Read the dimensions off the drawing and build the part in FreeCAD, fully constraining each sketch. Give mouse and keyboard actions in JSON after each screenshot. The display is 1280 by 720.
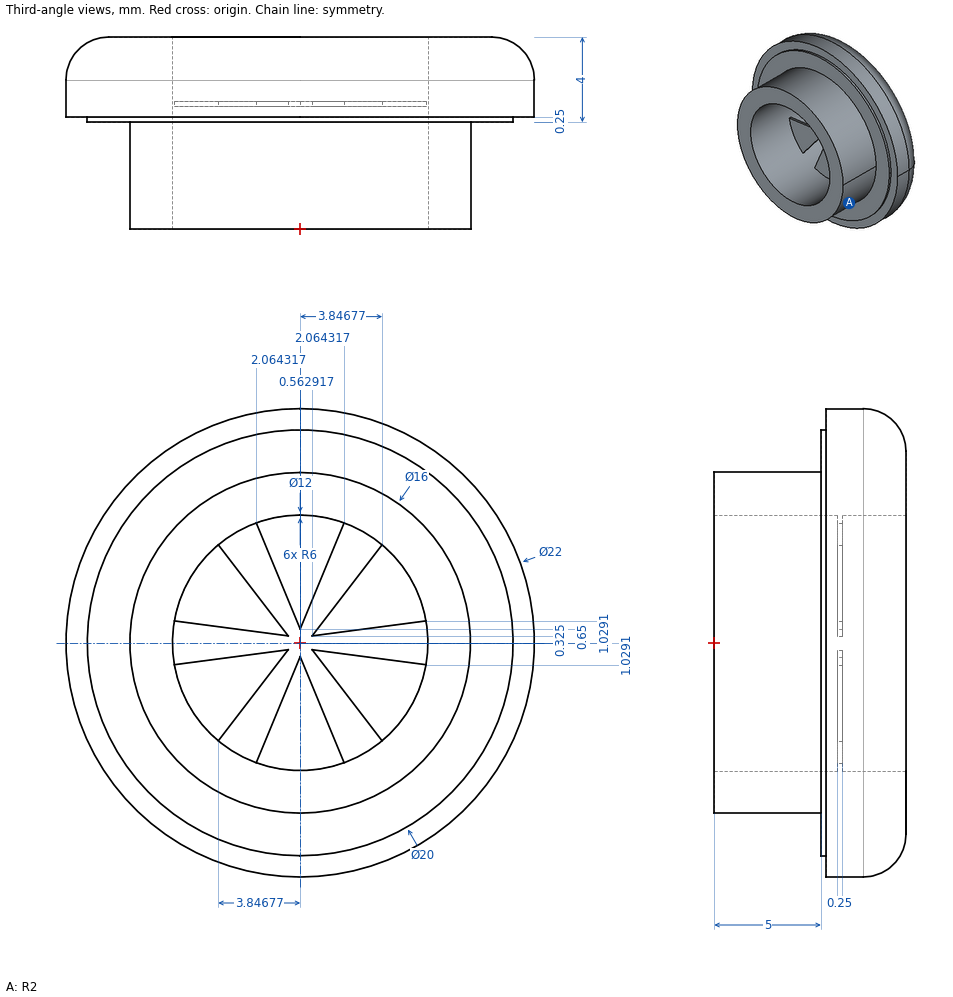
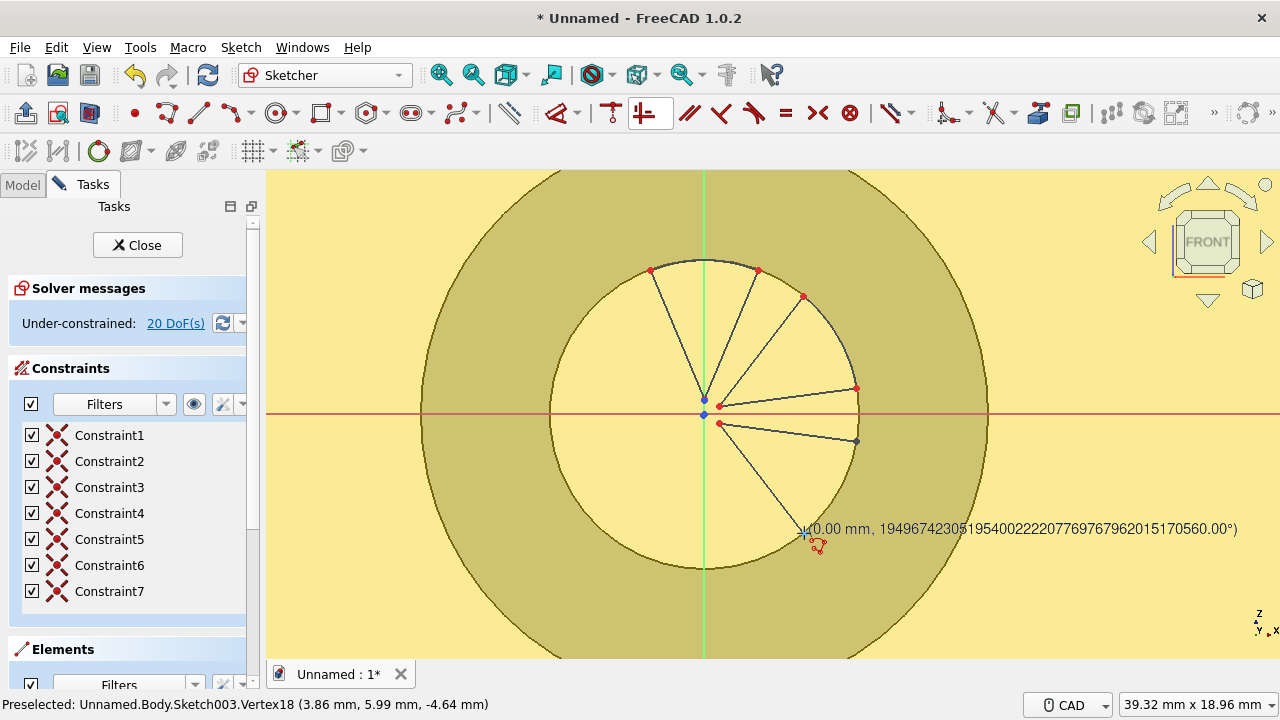
{"action": "key", "text": "g 3 a"}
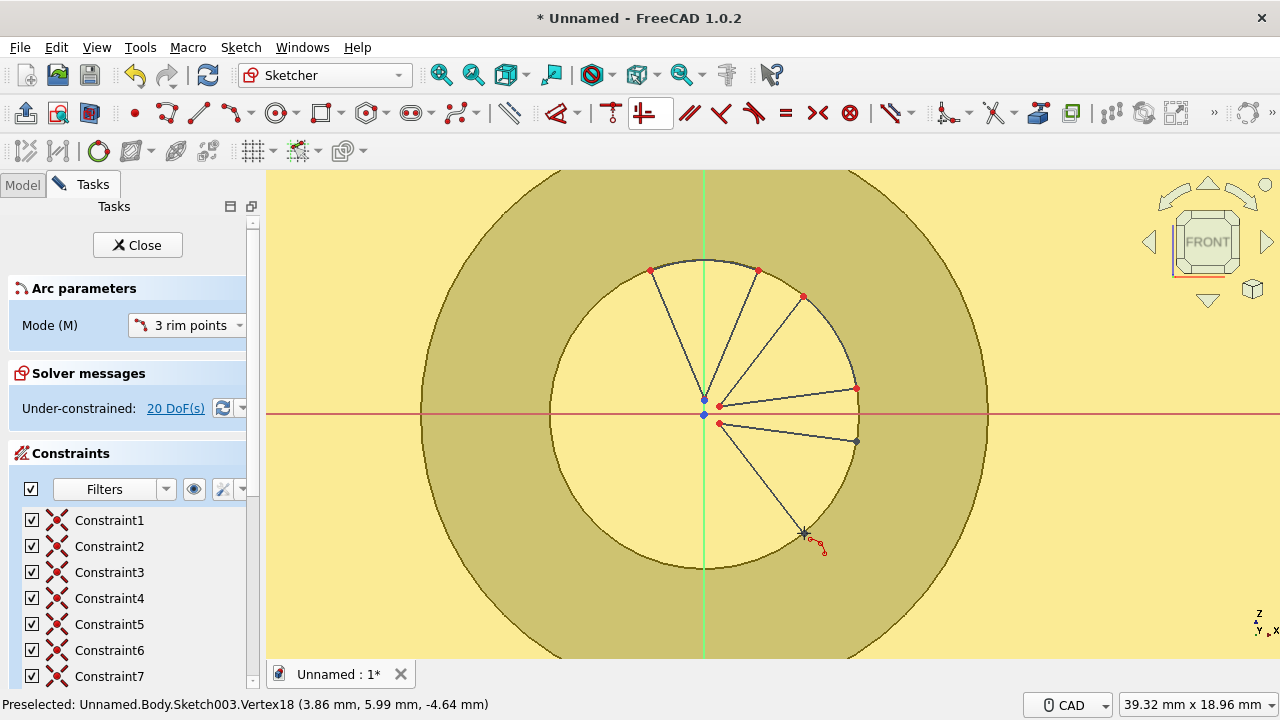
{"action": "left_click", "coordinate": [804, 534]}
{"action": "left_click", "coordinate": [857, 442]}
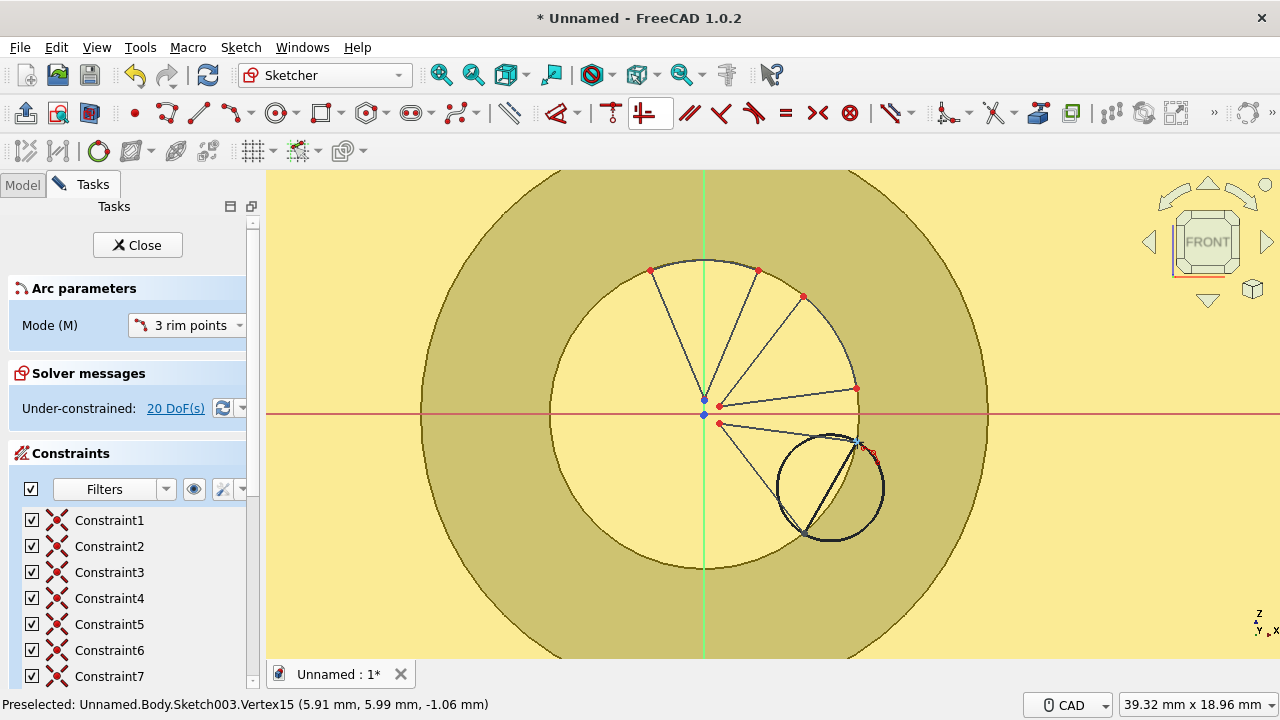
{"action": "scroll", "coordinate": [838, 492], "scroll_direction": "up", "scroll_amount": 3}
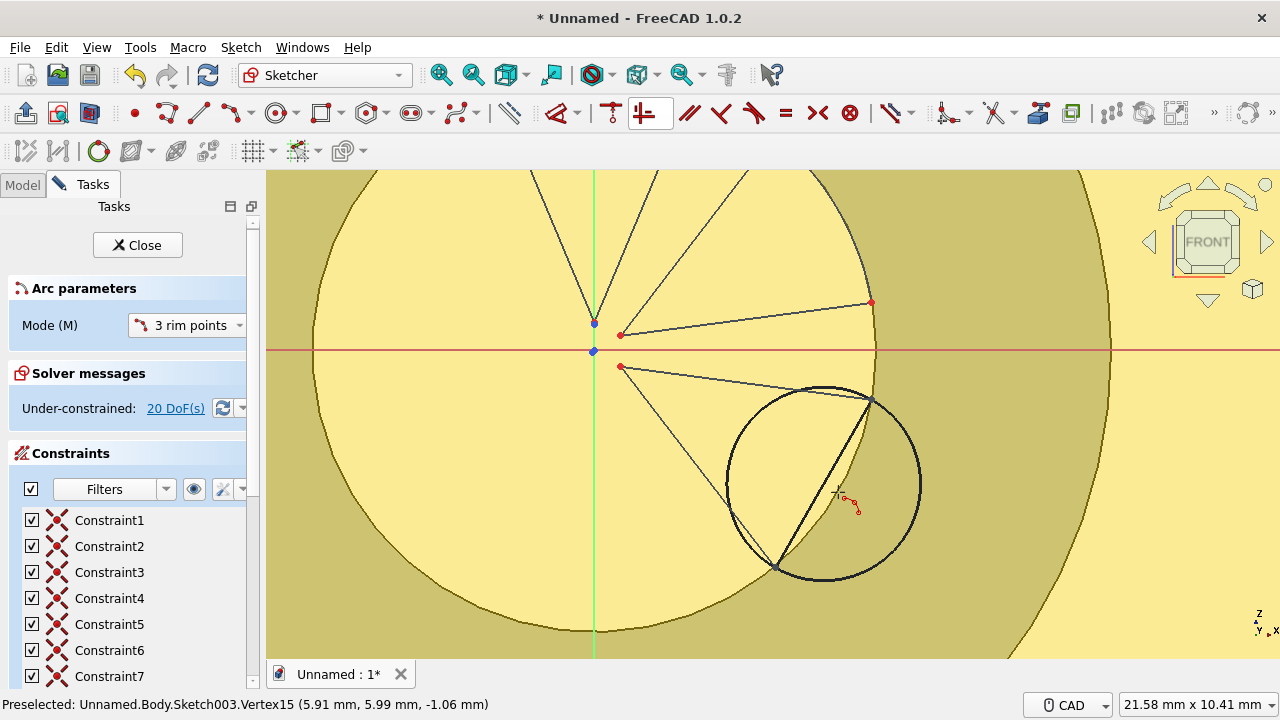
{"action": "left_click", "coordinate": [838, 491]}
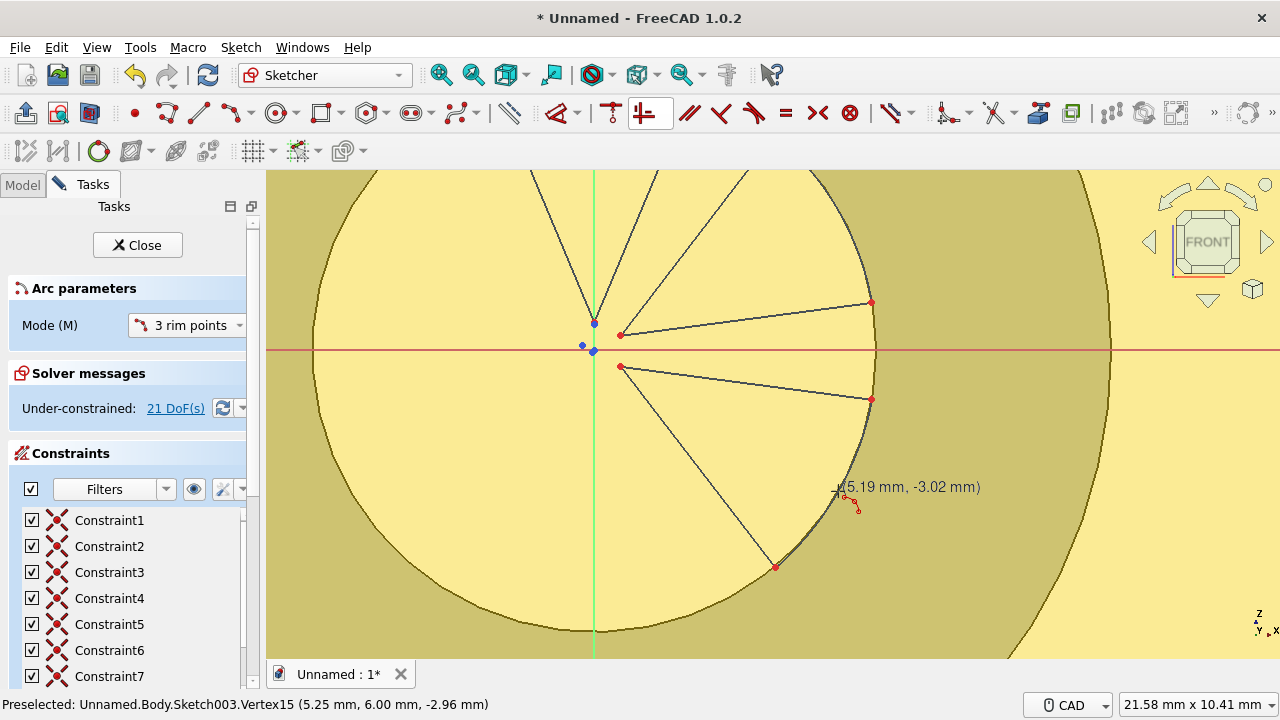
{"action": "left_click", "coordinate": [168, 114]}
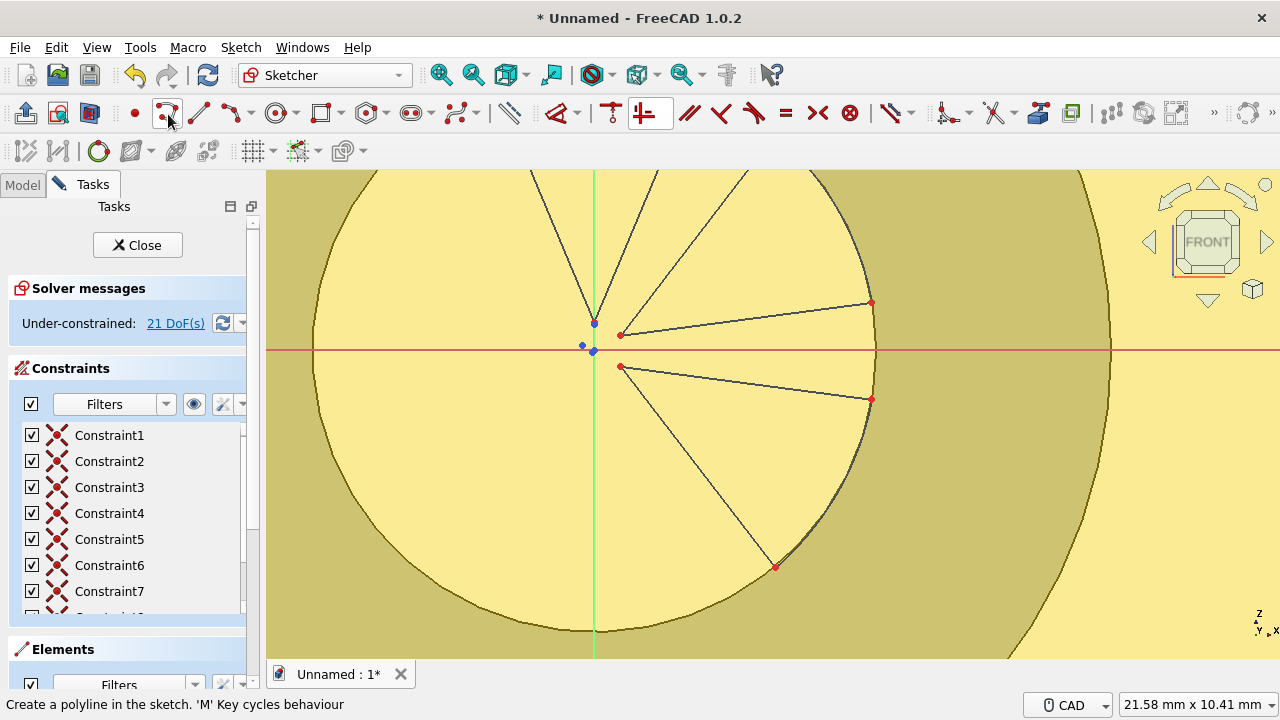
{"action": "left_click", "coordinate": [691, 615]}
{"action": "left_click", "coordinate": [594, 381]}
{"action": "left_click", "coordinate": [497, 615]}
{"action": "right_click", "coordinate": [497, 615]}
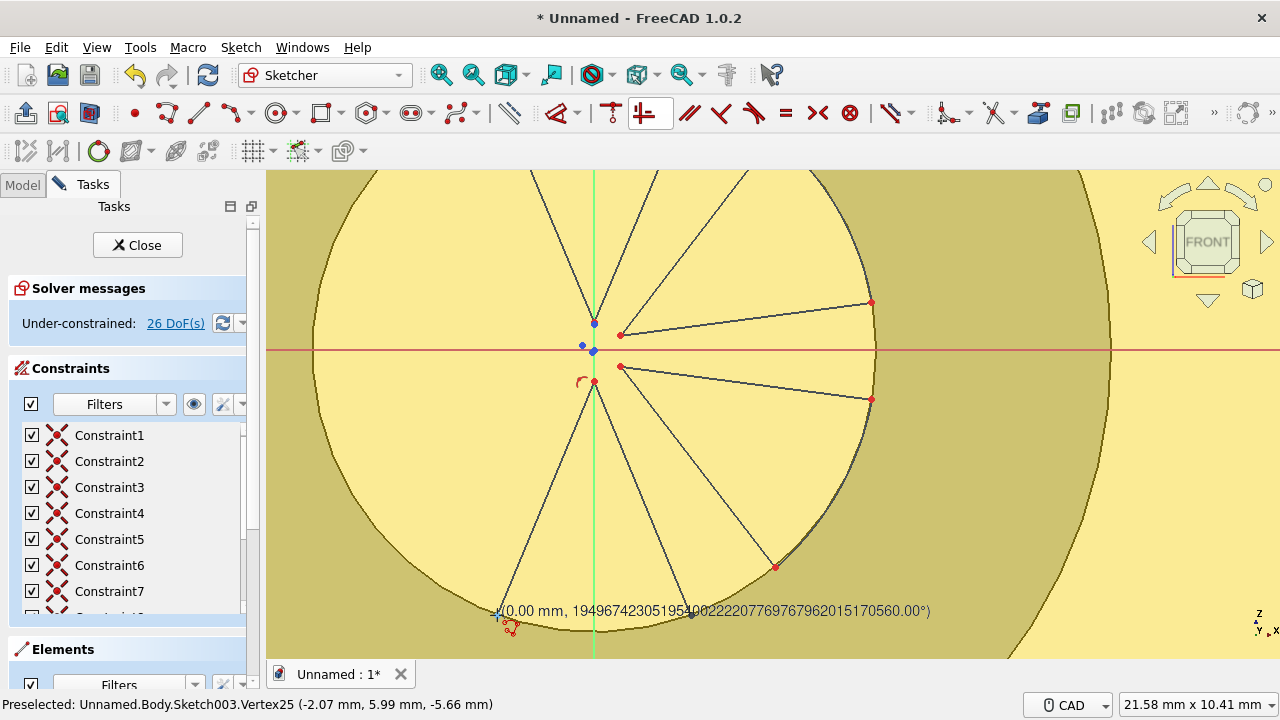
{"action": "left_click", "coordinate": [232, 114]}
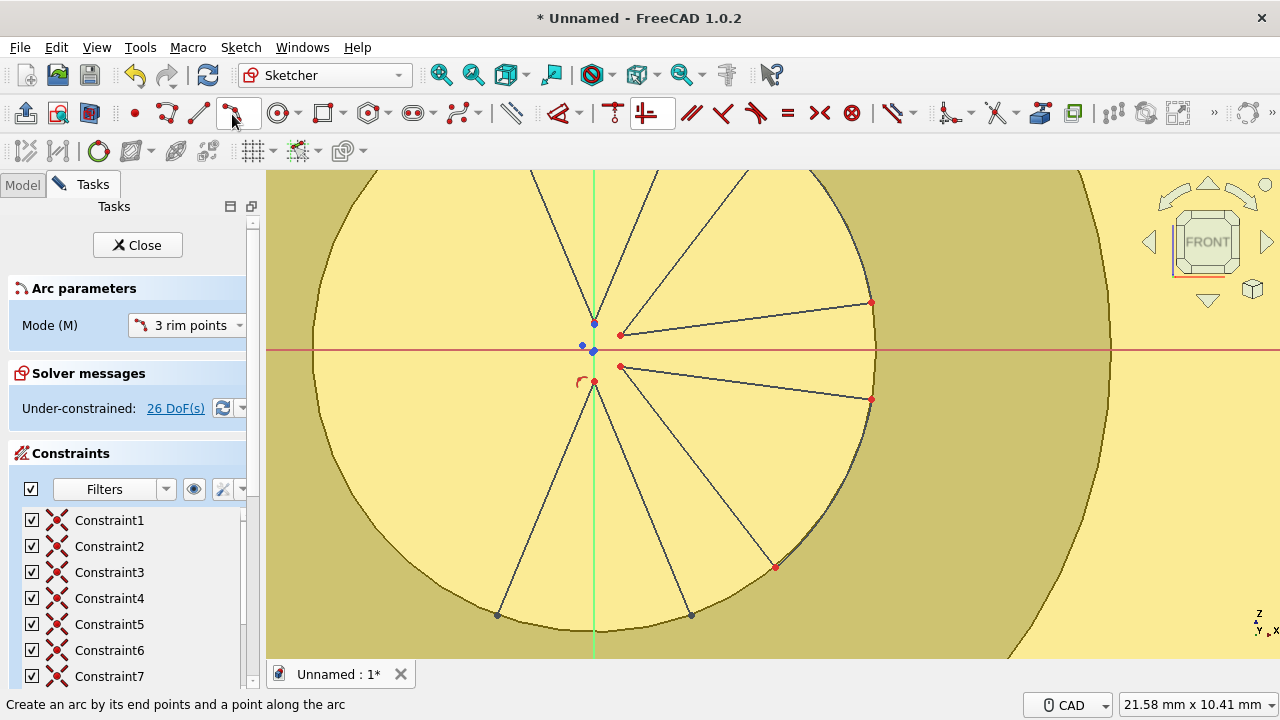
{"action": "left_click", "coordinate": [497, 616]}
{"action": "left_click", "coordinate": [691, 616]}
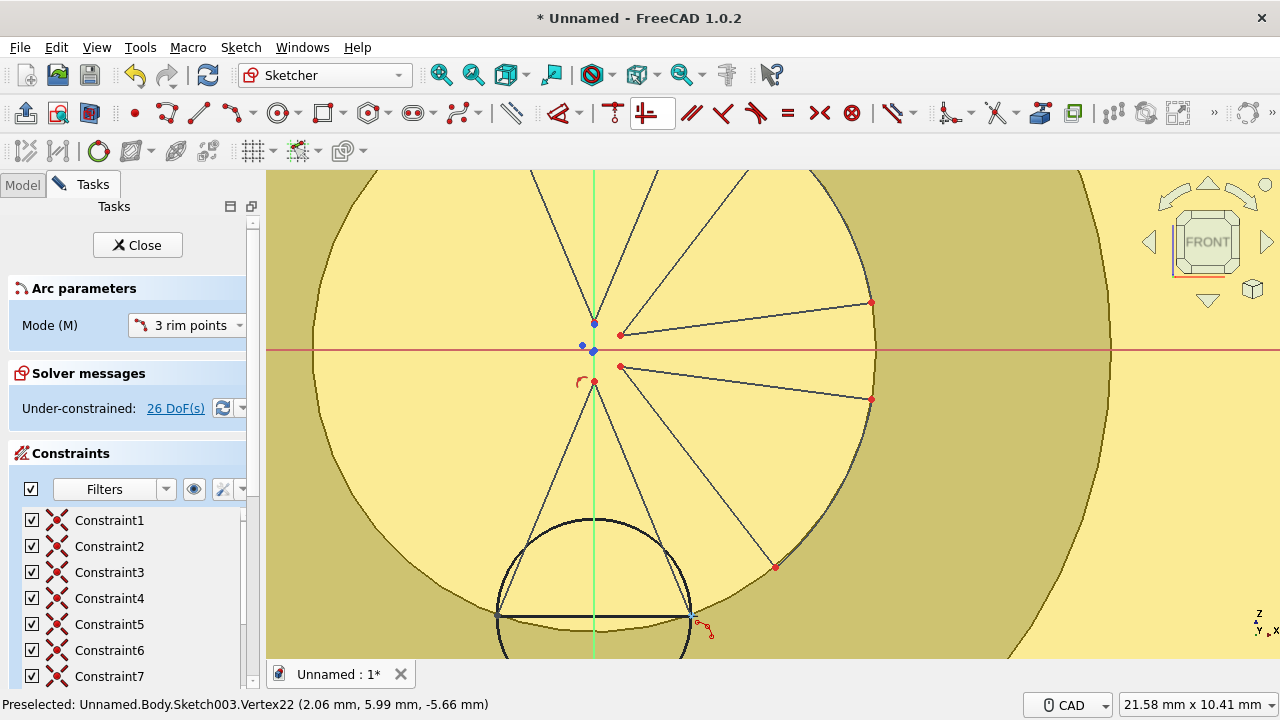
{"action": "scroll", "coordinate": [839, 493], "scroll_direction": "down", "scroll_amount": 3}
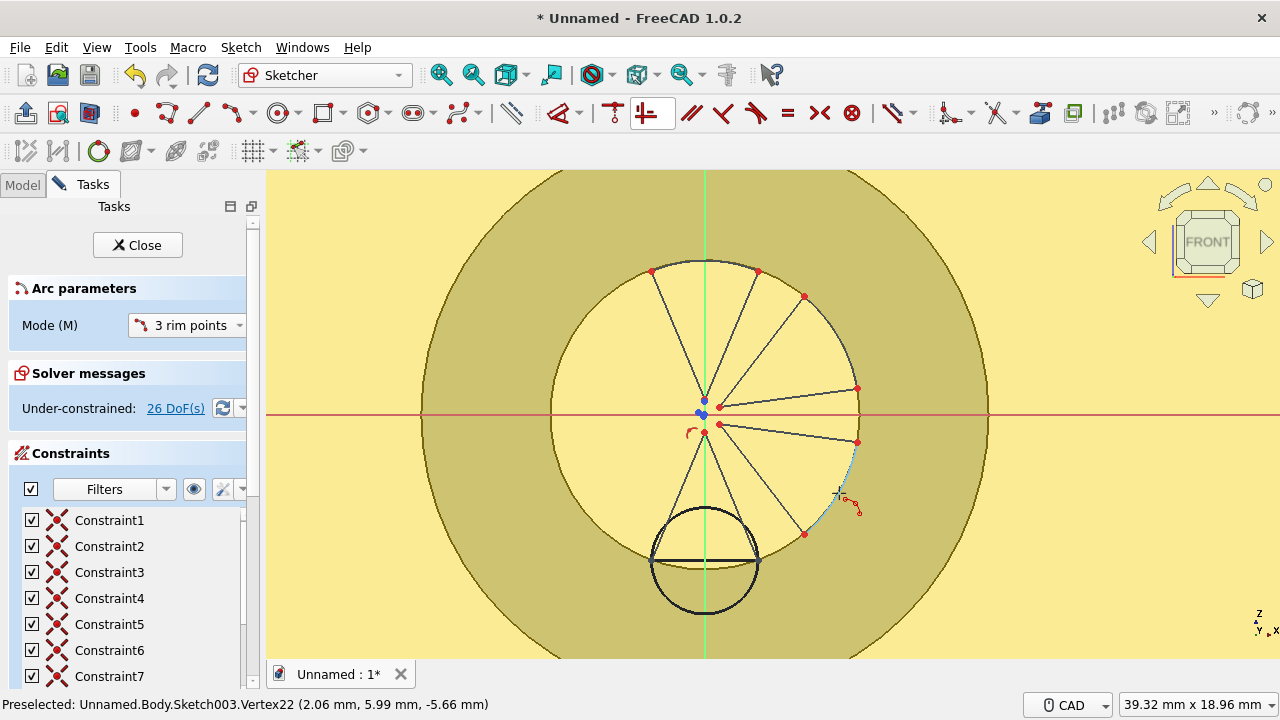
{"action": "scroll", "coordinate": [694, 569], "scroll_direction": "up", "scroll_amount": 3}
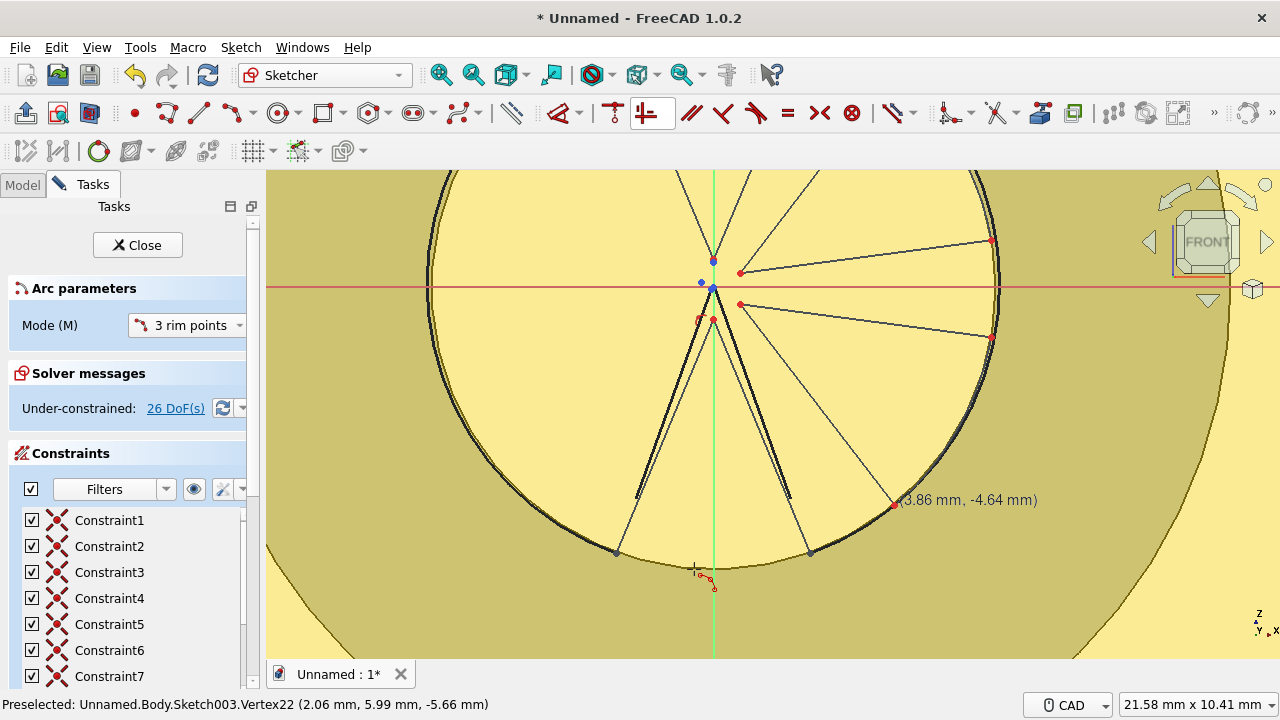
{"action": "left_click", "coordinate": [694, 569]}